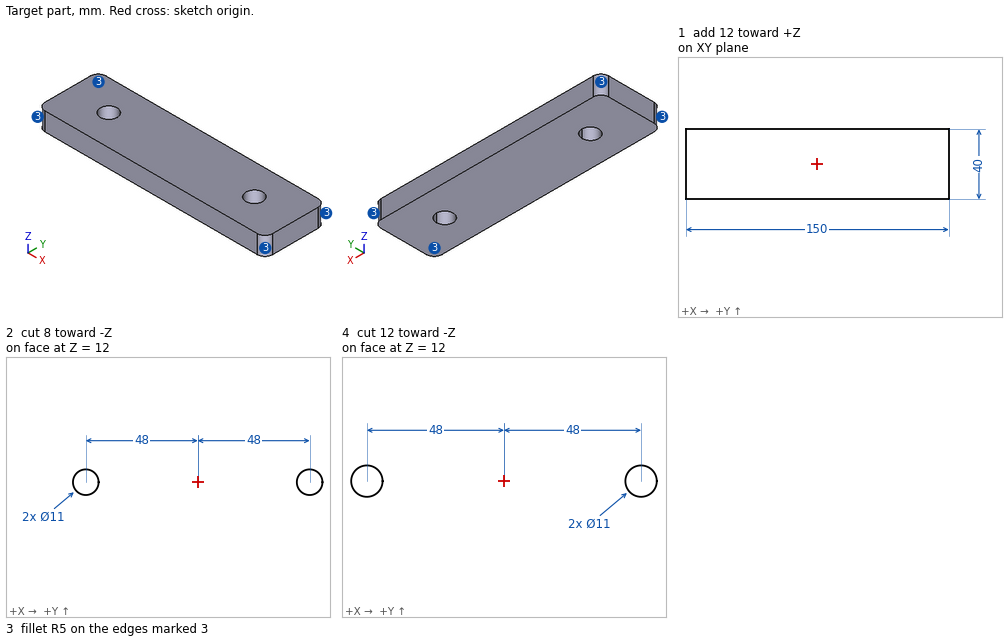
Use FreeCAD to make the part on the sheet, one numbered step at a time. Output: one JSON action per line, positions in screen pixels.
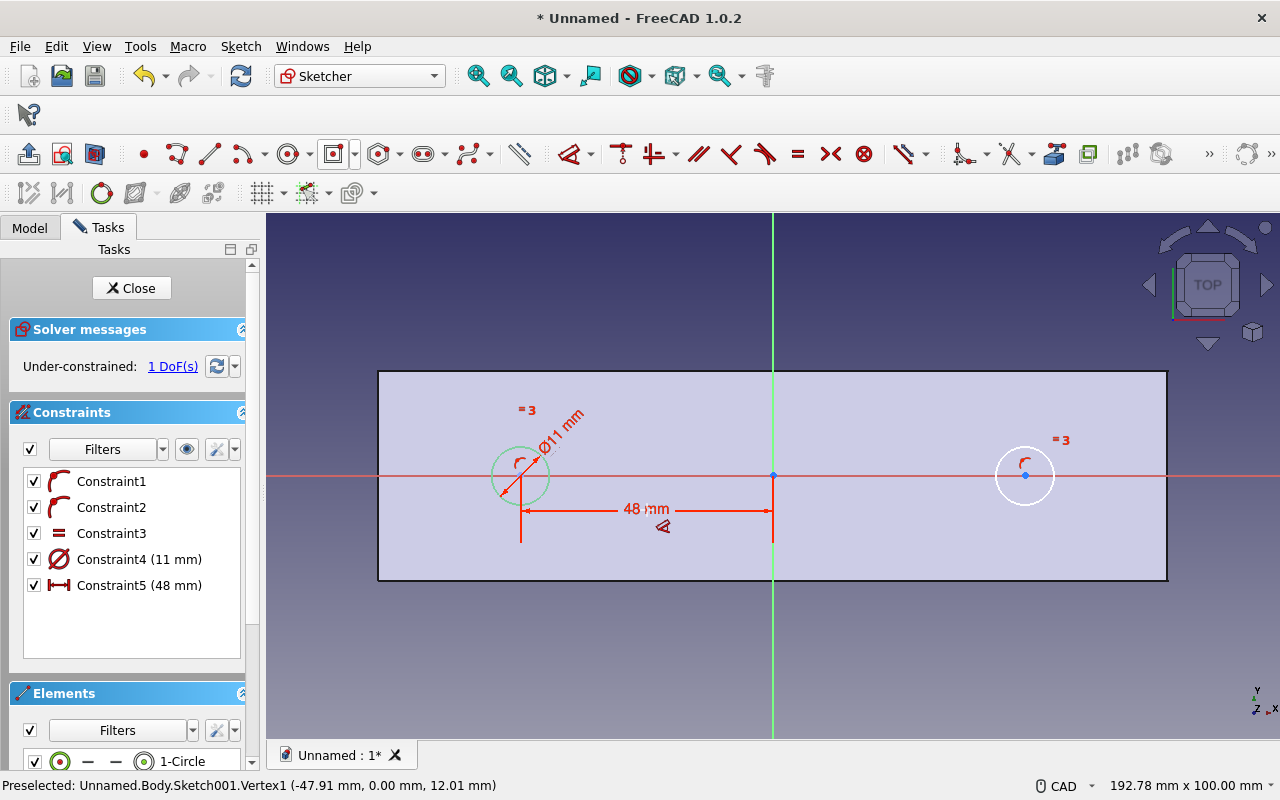
{"action": "left_click", "coordinate": [1025, 476]}
{"action": "left_click", "coordinate": [899, 510]}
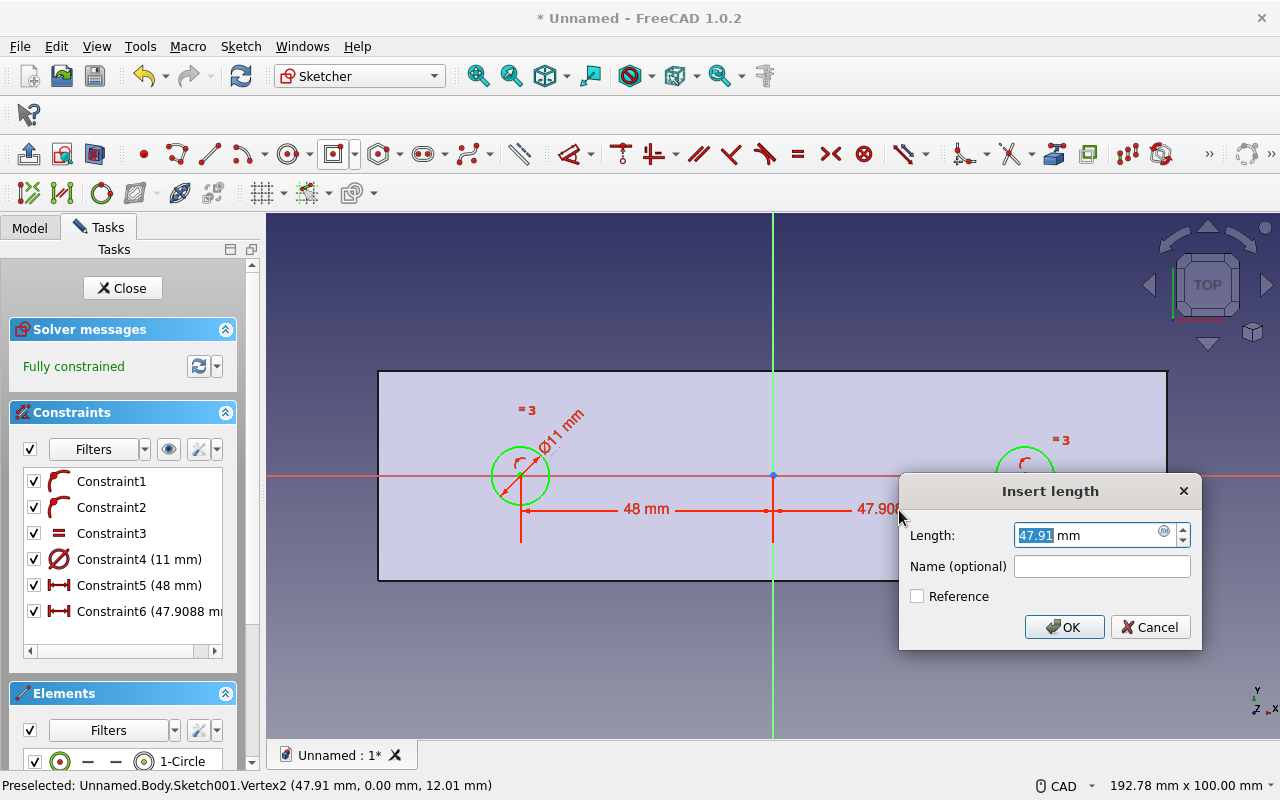
{"action": "type", "text": "48"}
{"action": "key", "text": "Return"}
{"action": "key", "text": "Escape"}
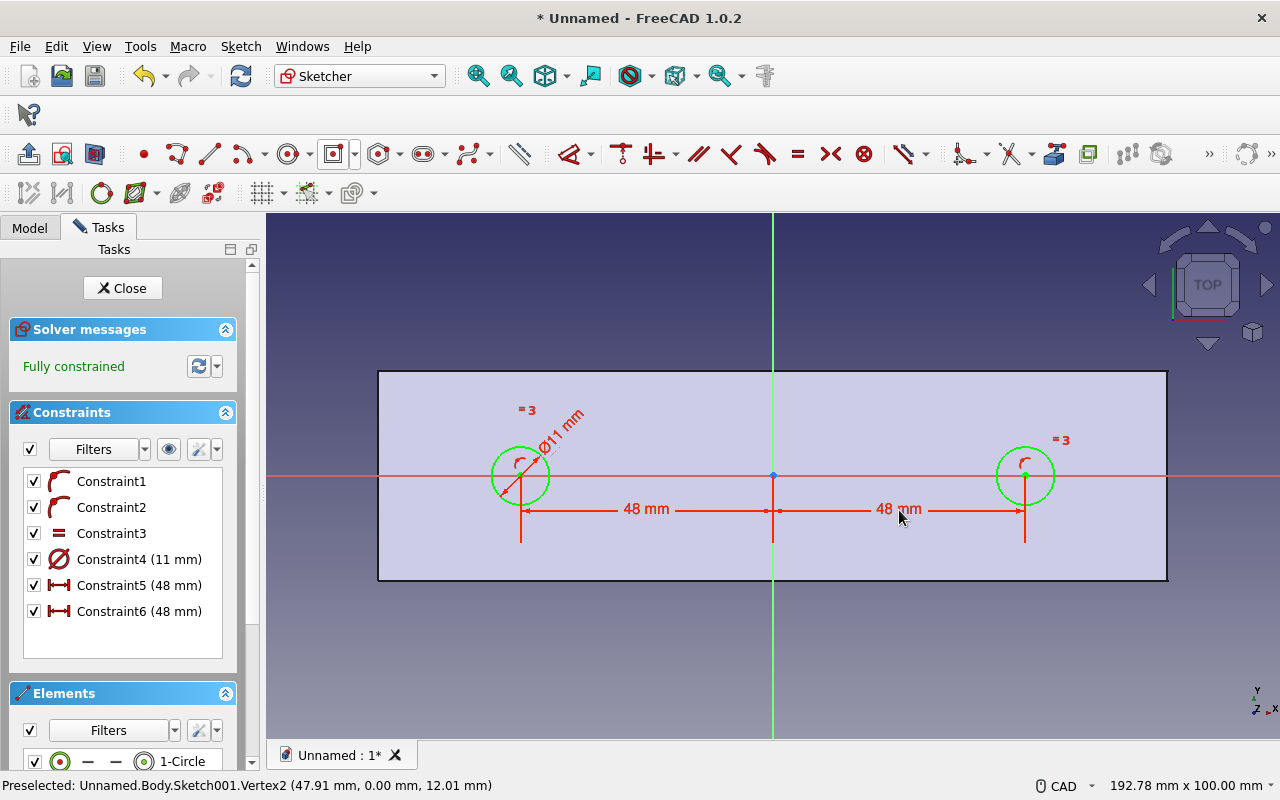
{"action": "left_click", "coordinate": [123, 288]}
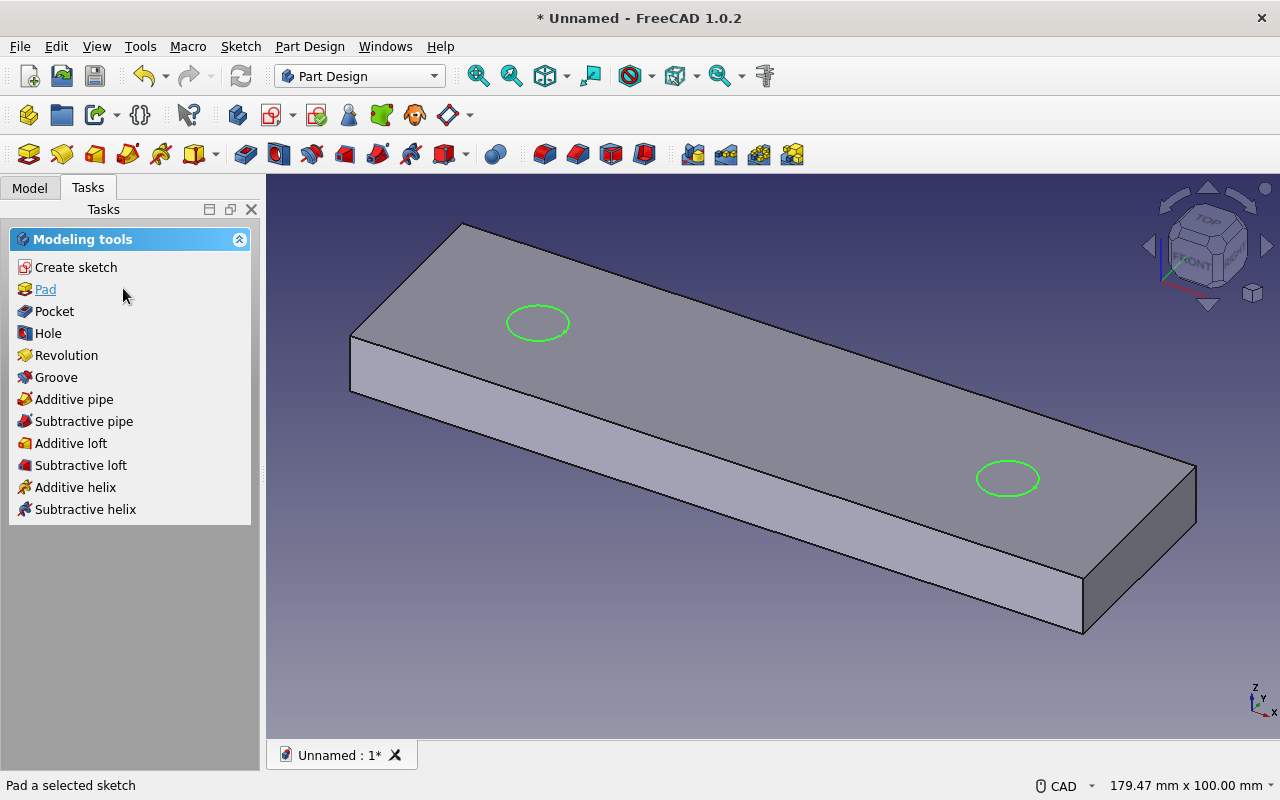
{"action": "left_click", "coordinate": [246, 154]}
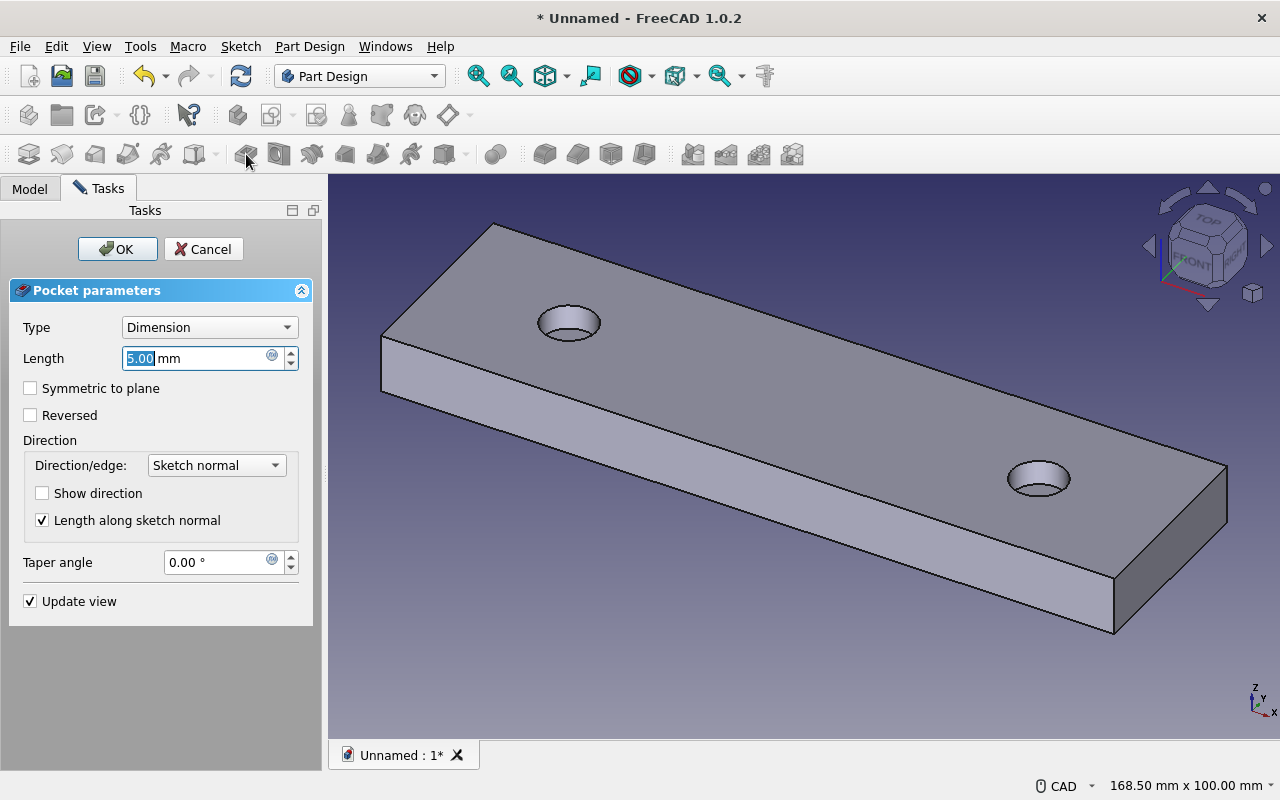
{"action": "type", "text": "8"}
{"action": "key", "text": "Tab"}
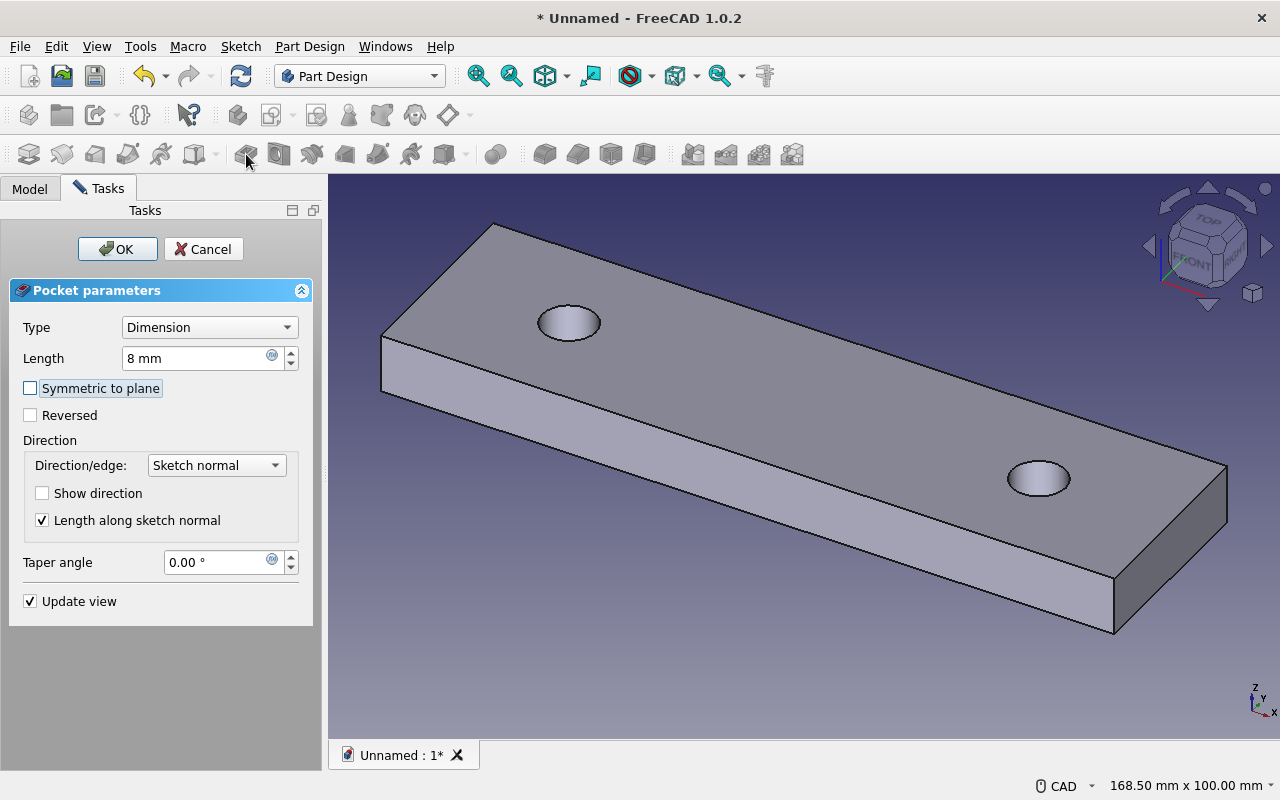
{"action": "left_click", "coordinate": [118, 249]}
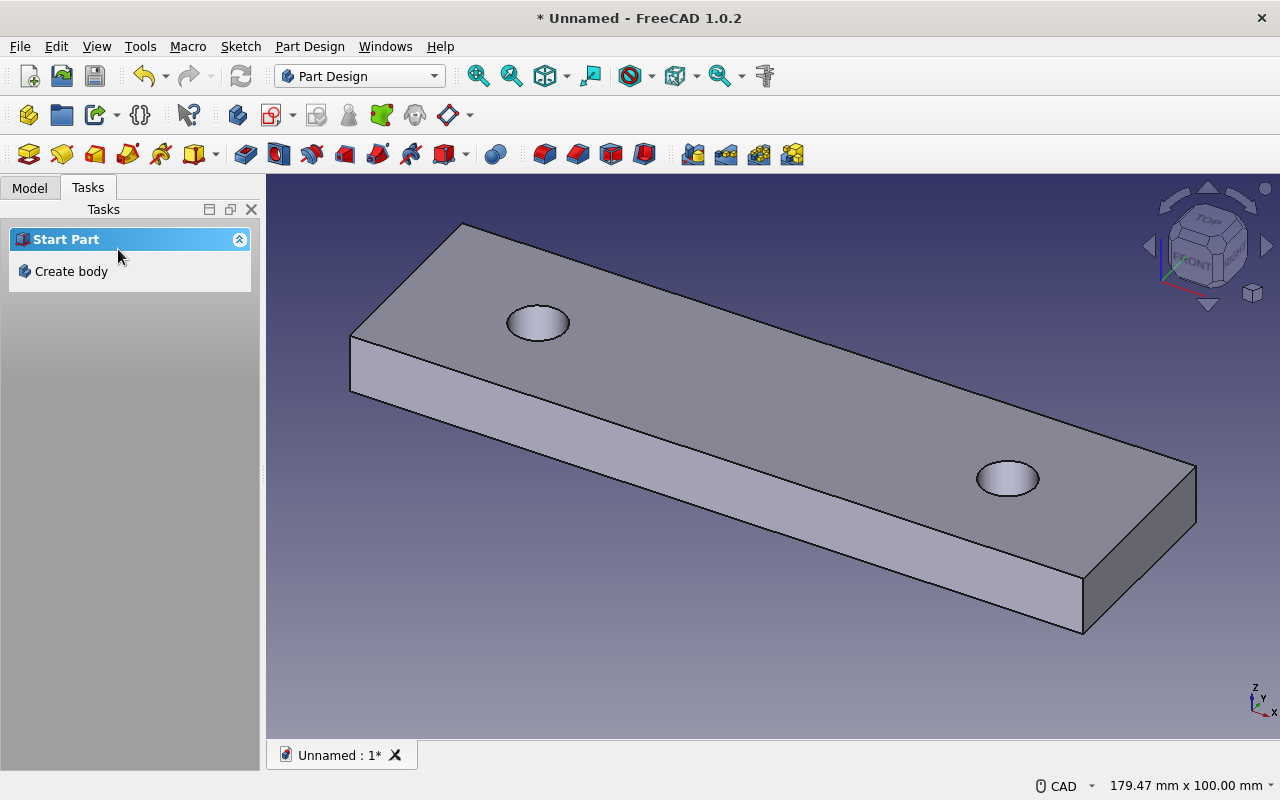
{"action": "left_click", "coordinate": [1083, 605]}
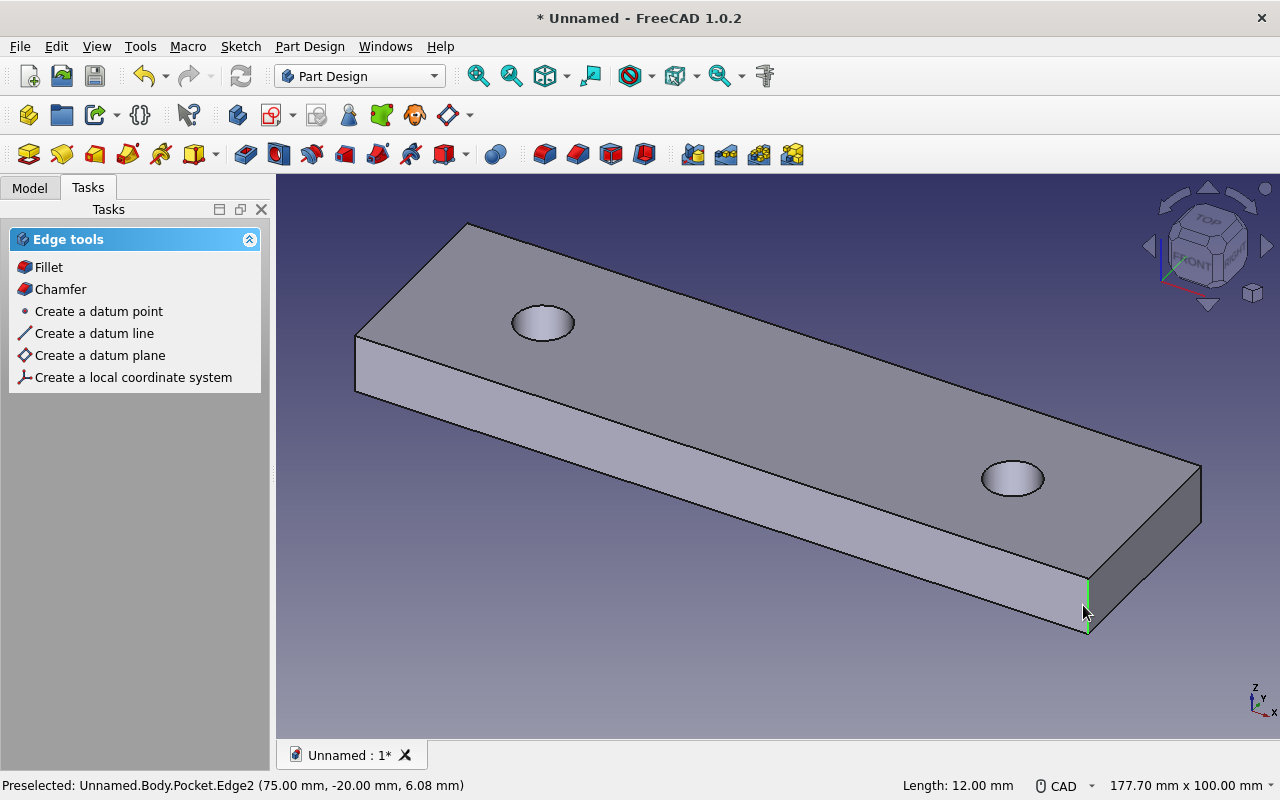
{"action": "key", "text": "0"}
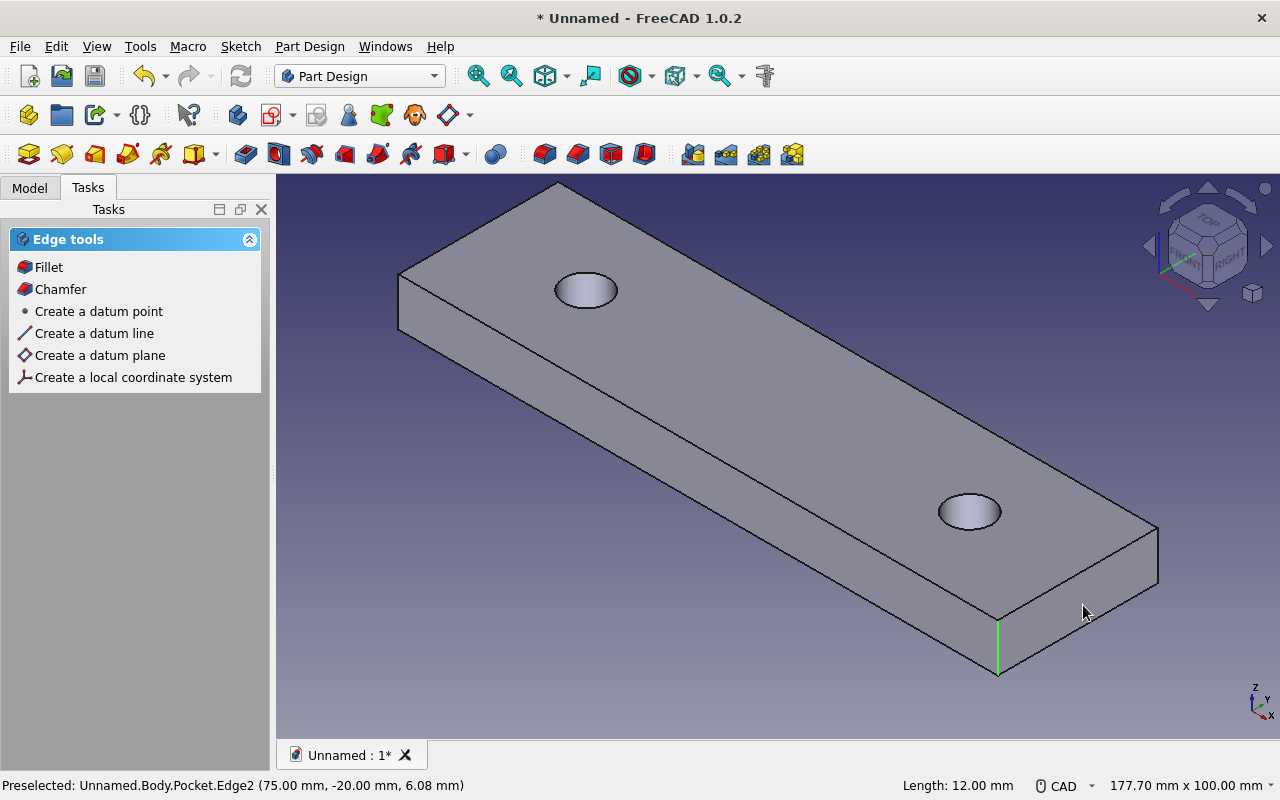
{"action": "key", "text": "2"}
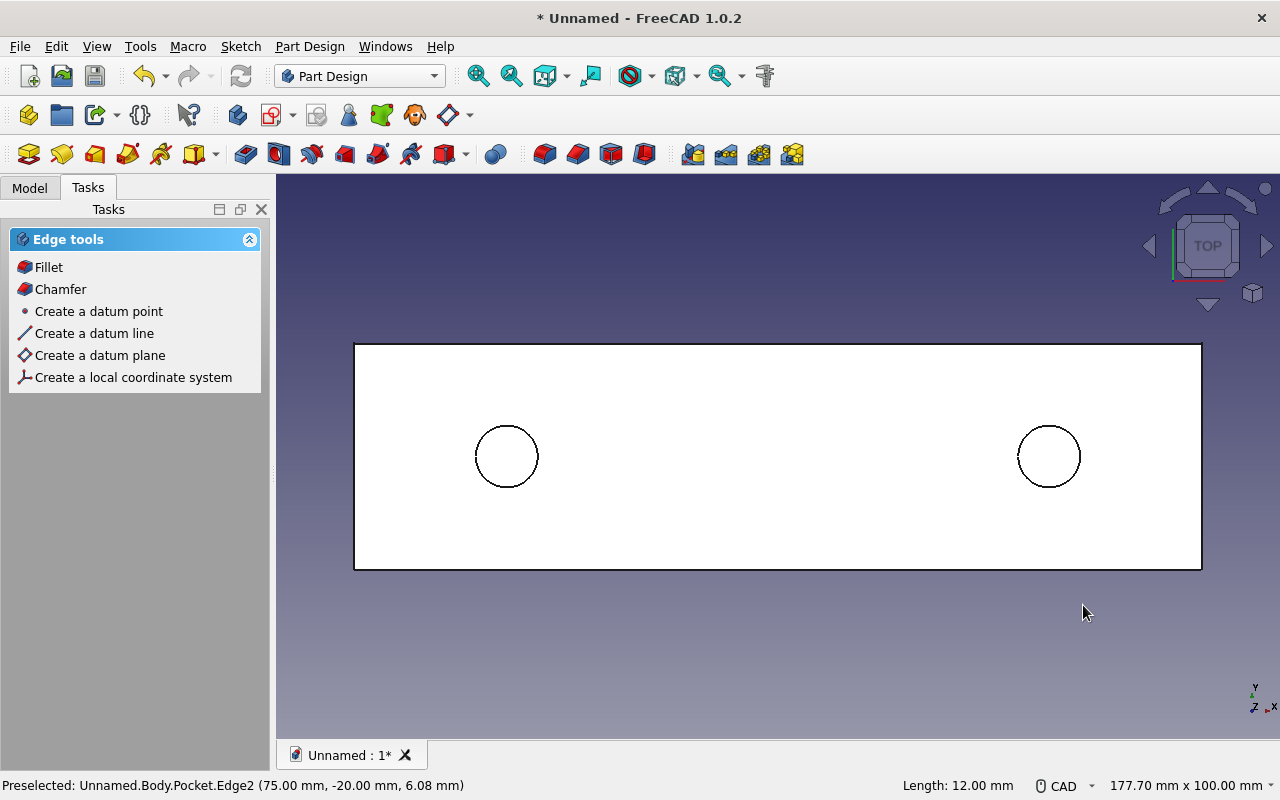
{"action": "key", "text": "1"}